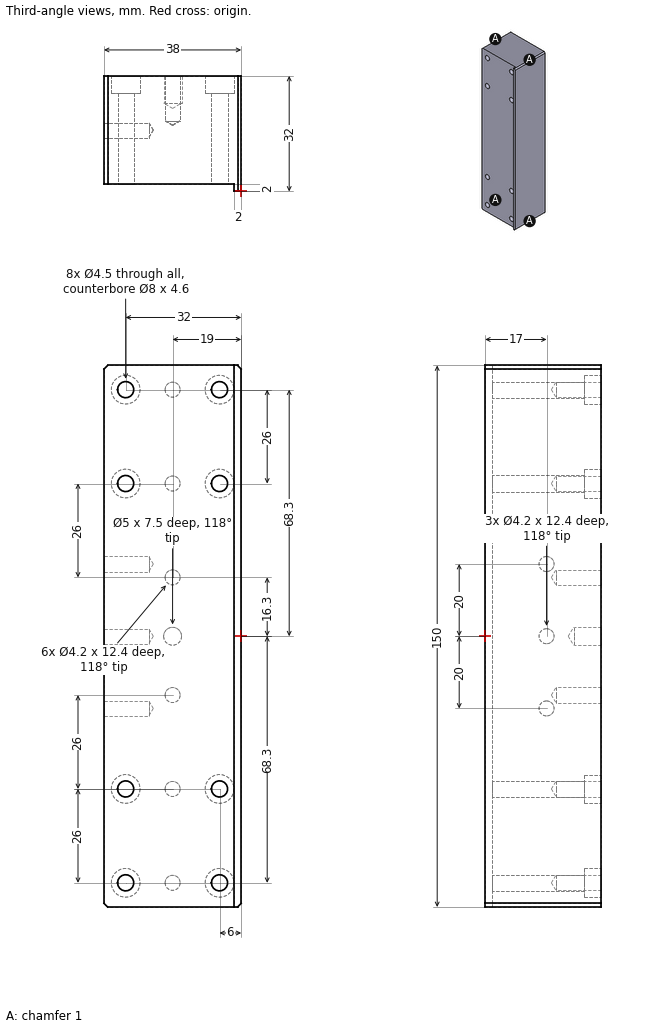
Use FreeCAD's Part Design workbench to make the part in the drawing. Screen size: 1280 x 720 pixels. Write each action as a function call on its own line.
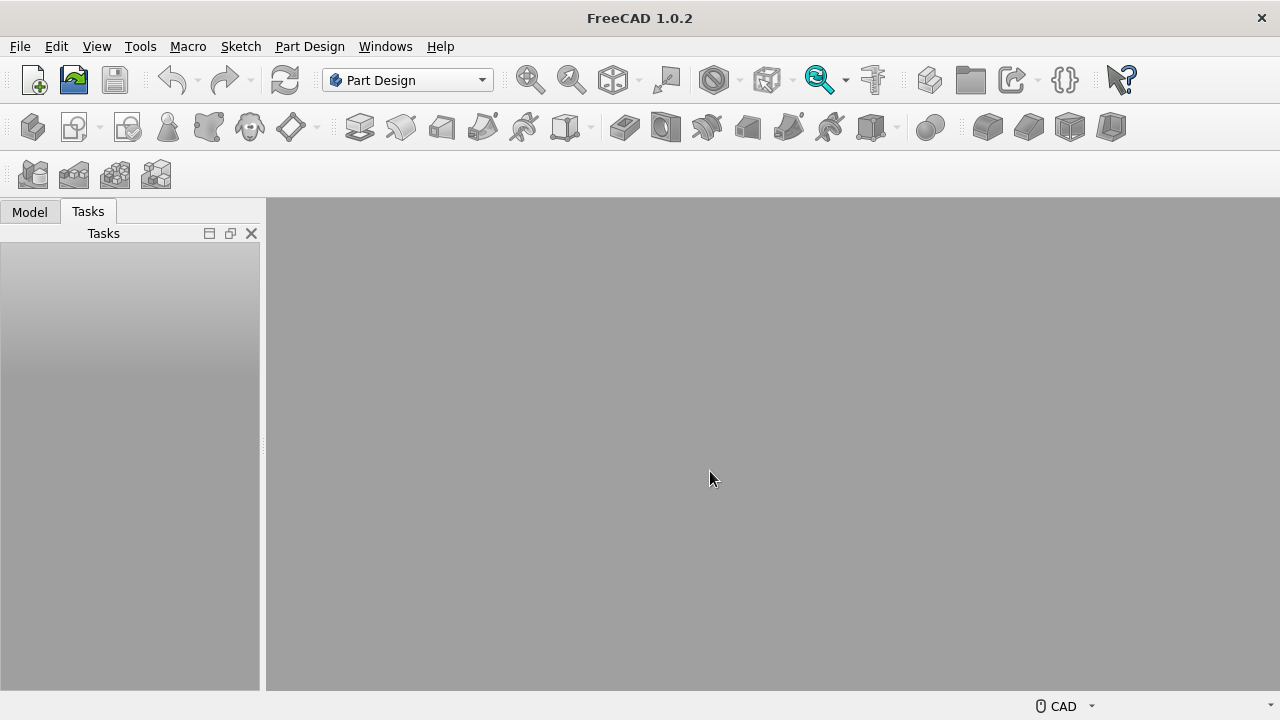
click(33, 80)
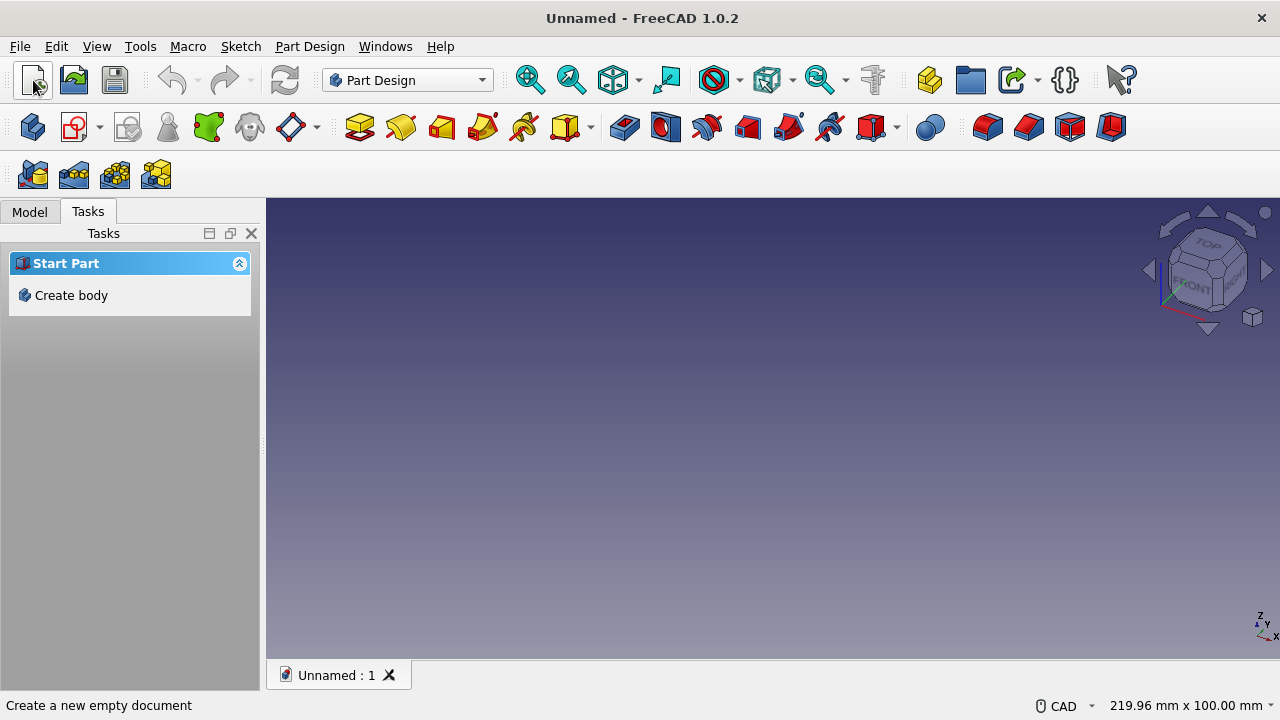
click(74, 128)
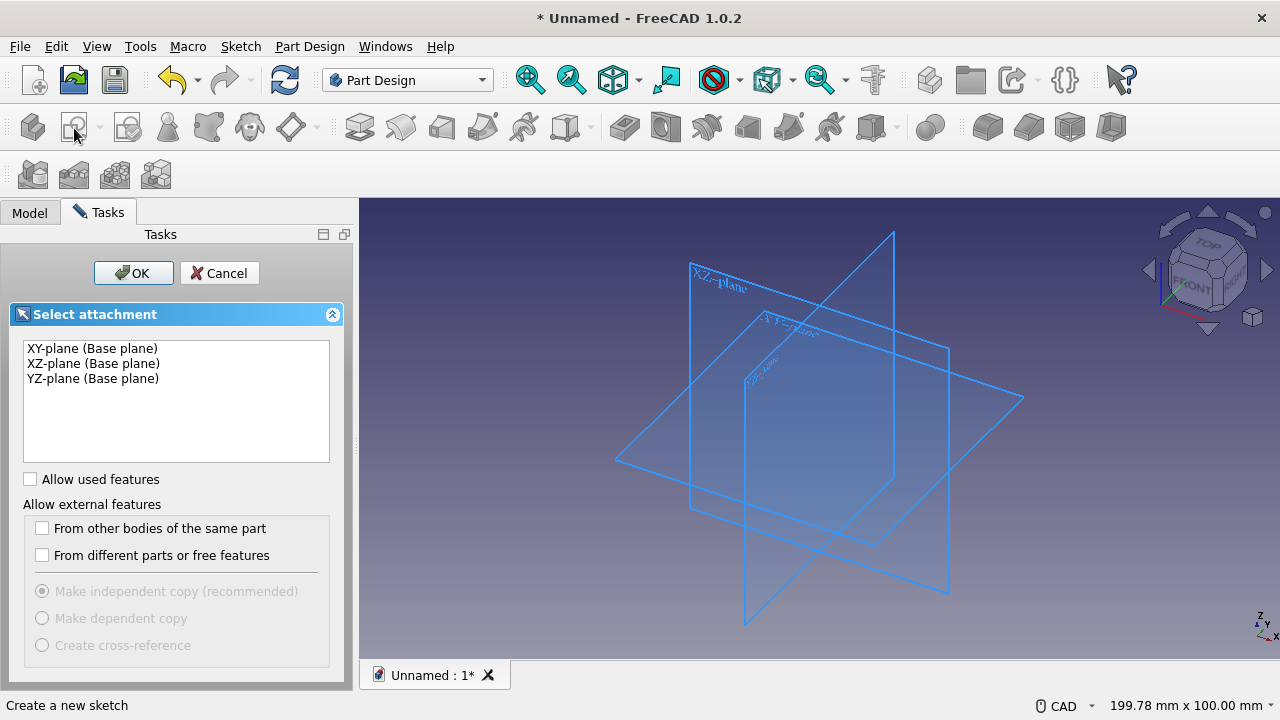
click(84, 348)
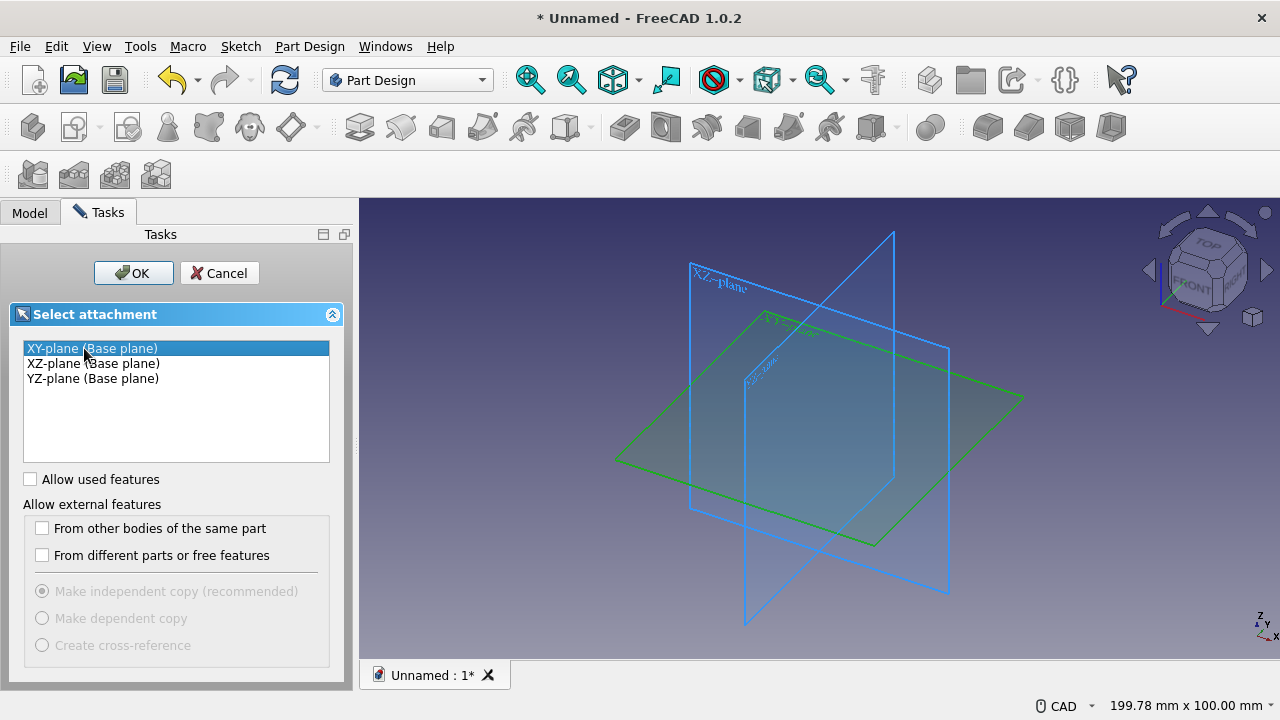
click(134, 273)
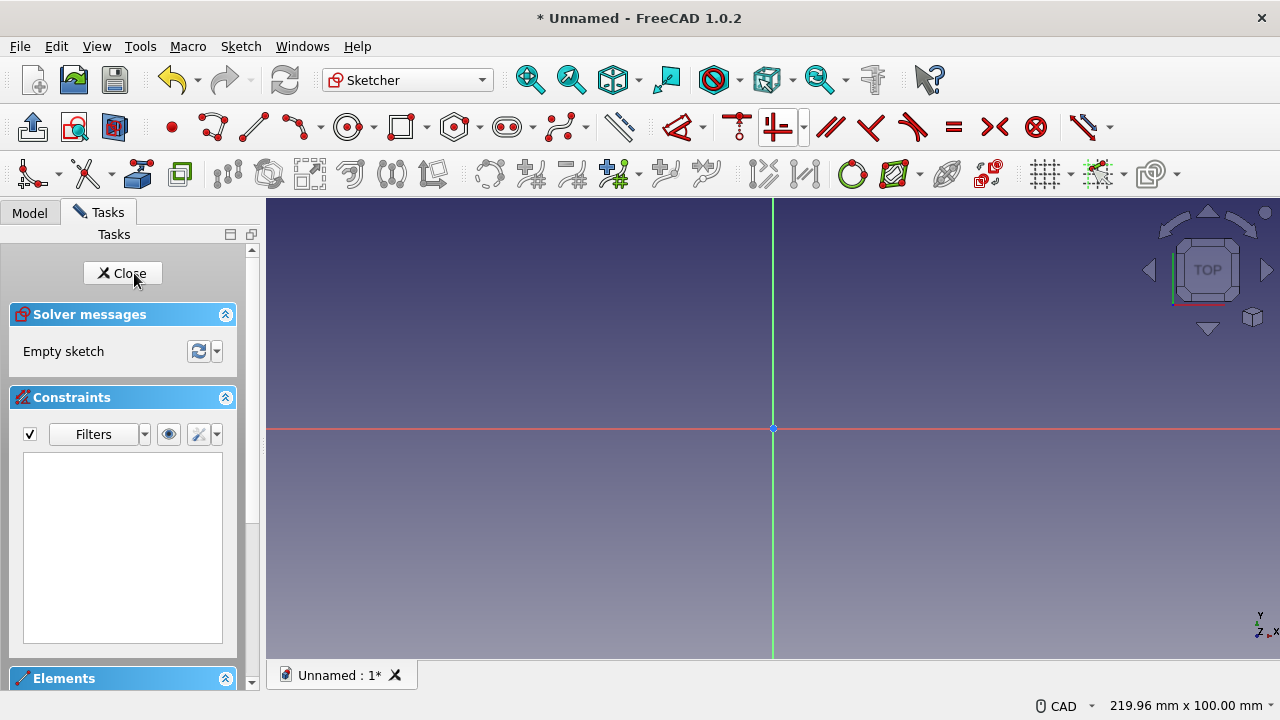
scroll(662, 265, up, 3)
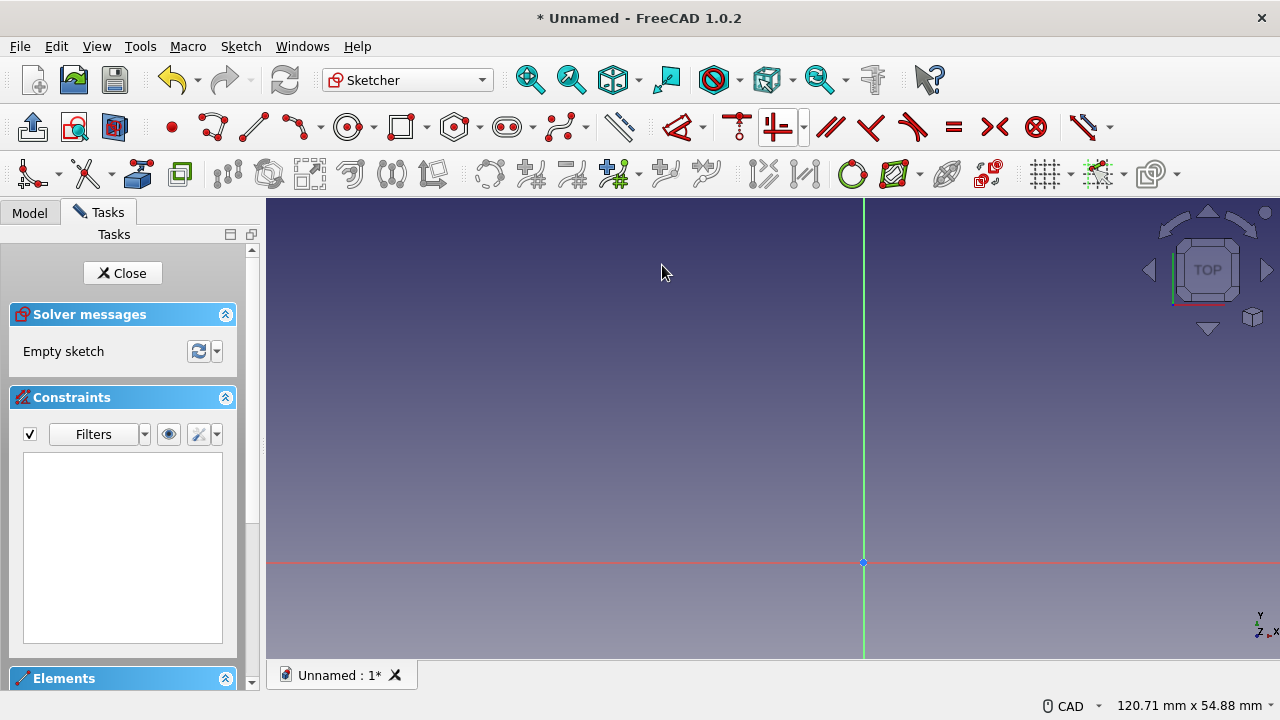
click(213, 128)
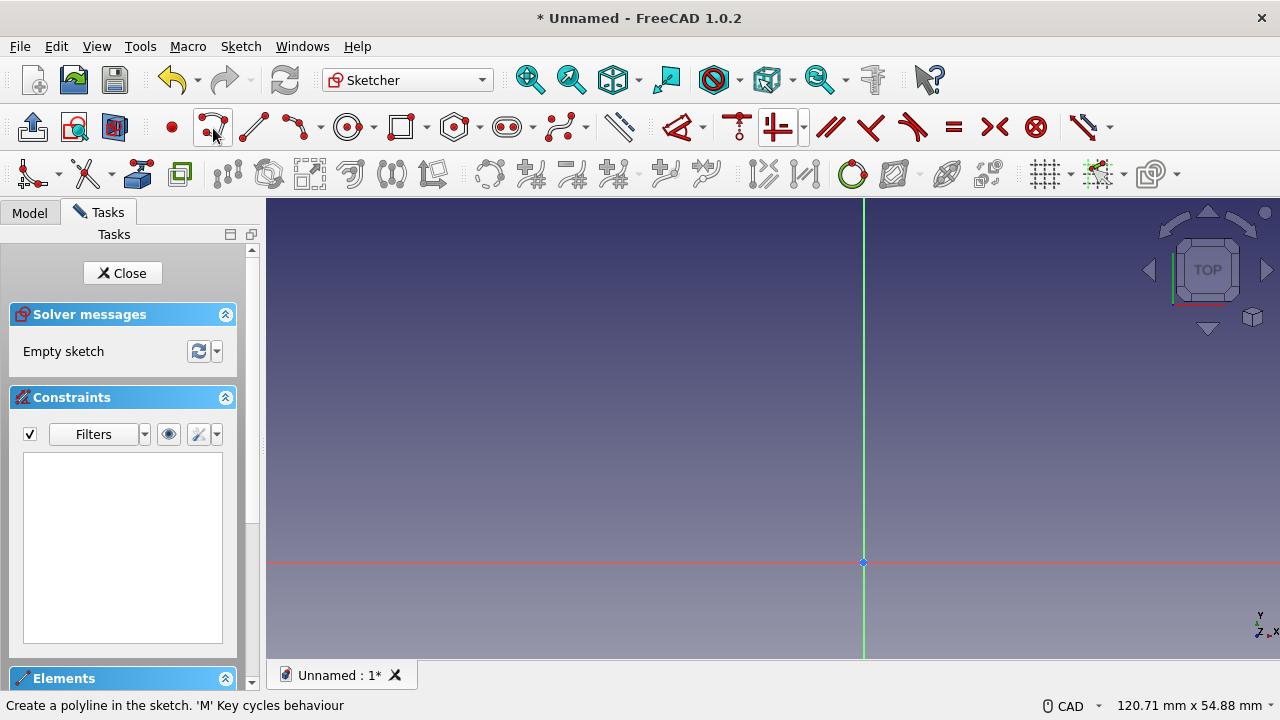
click(864, 563)
click(855, 294)
click(545, 294)
click(545, 546)
click(847, 546)
click(847, 554)
click(864, 563)
key(Escape)
key(Escape)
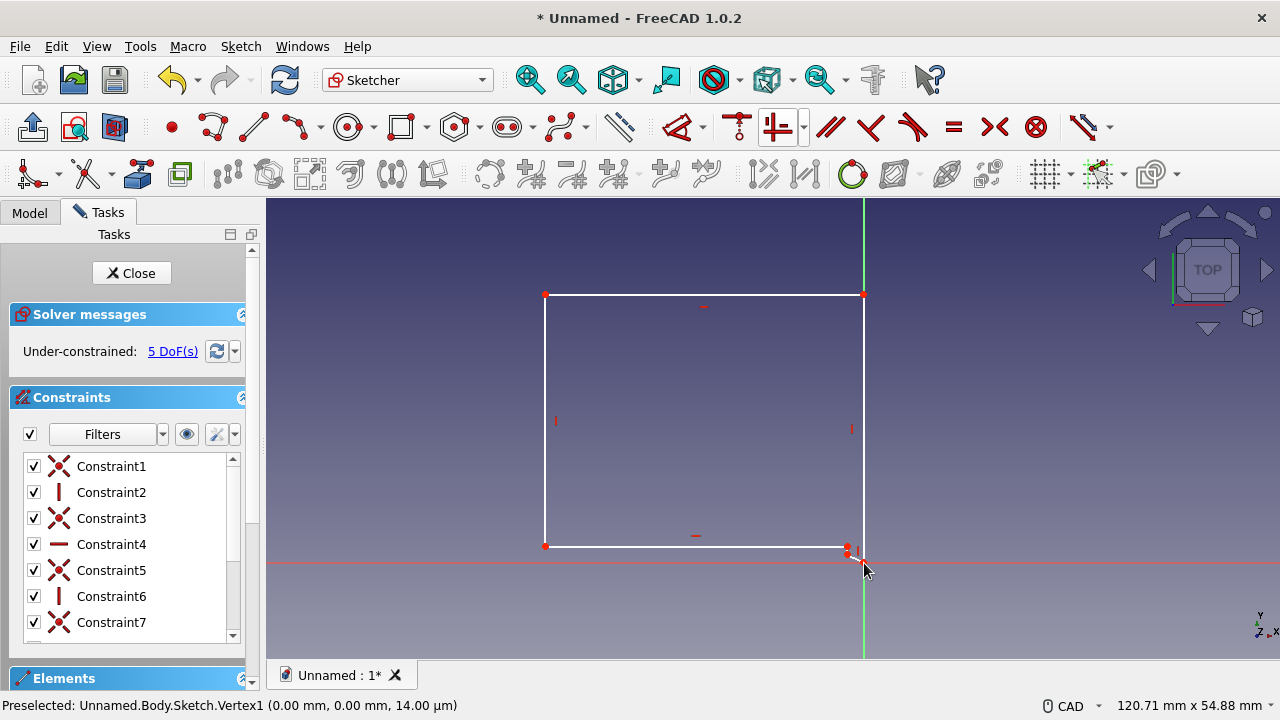
scroll(855, 559, up, 3)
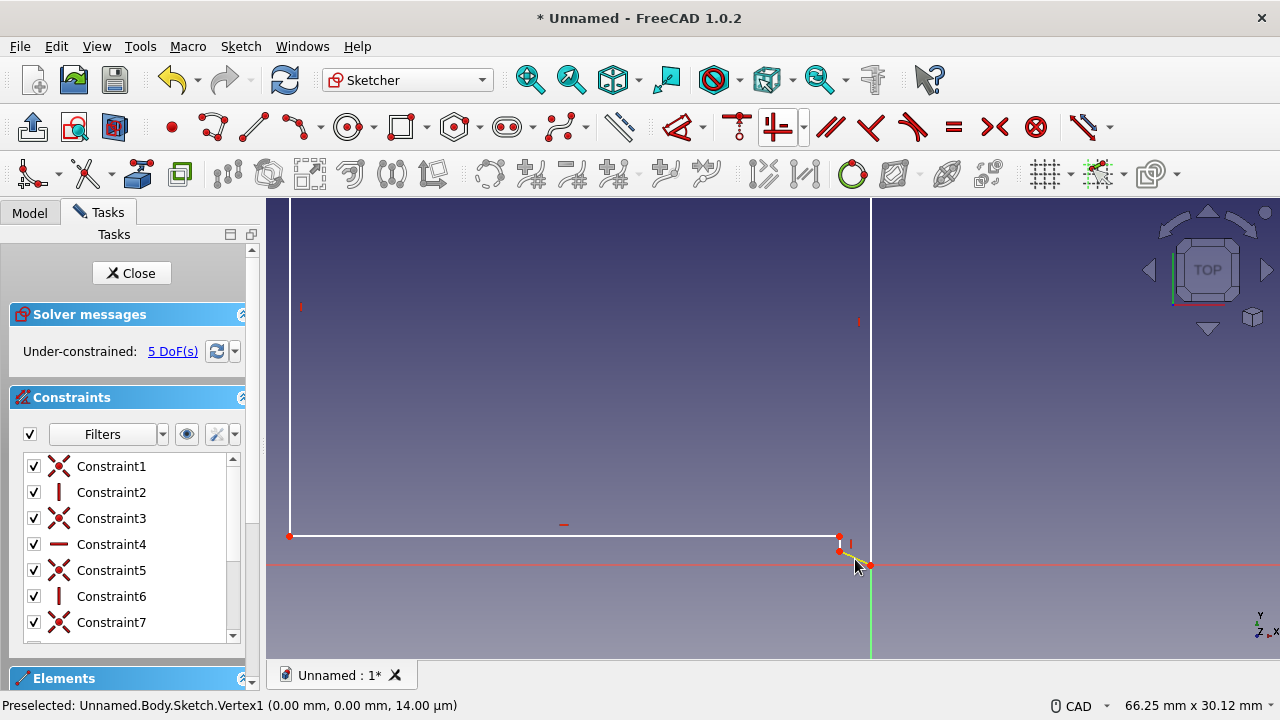
click(855, 558)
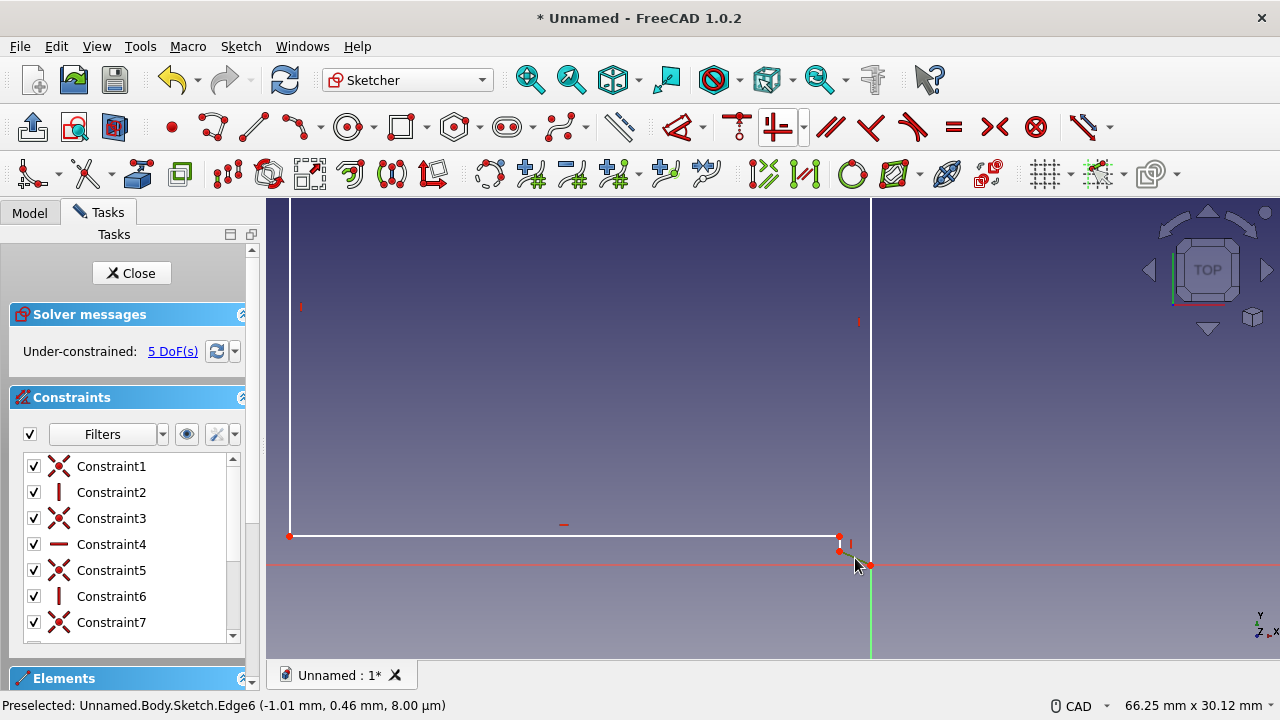
click(804, 128)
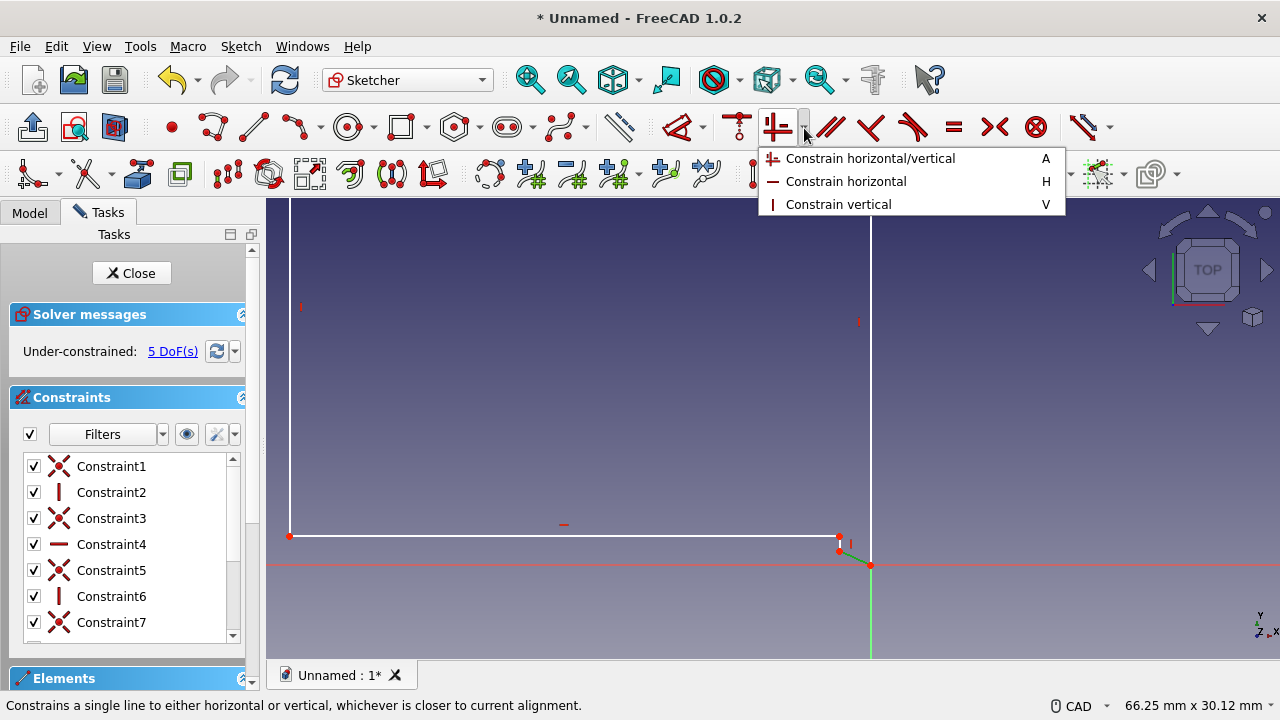
click(912, 182)